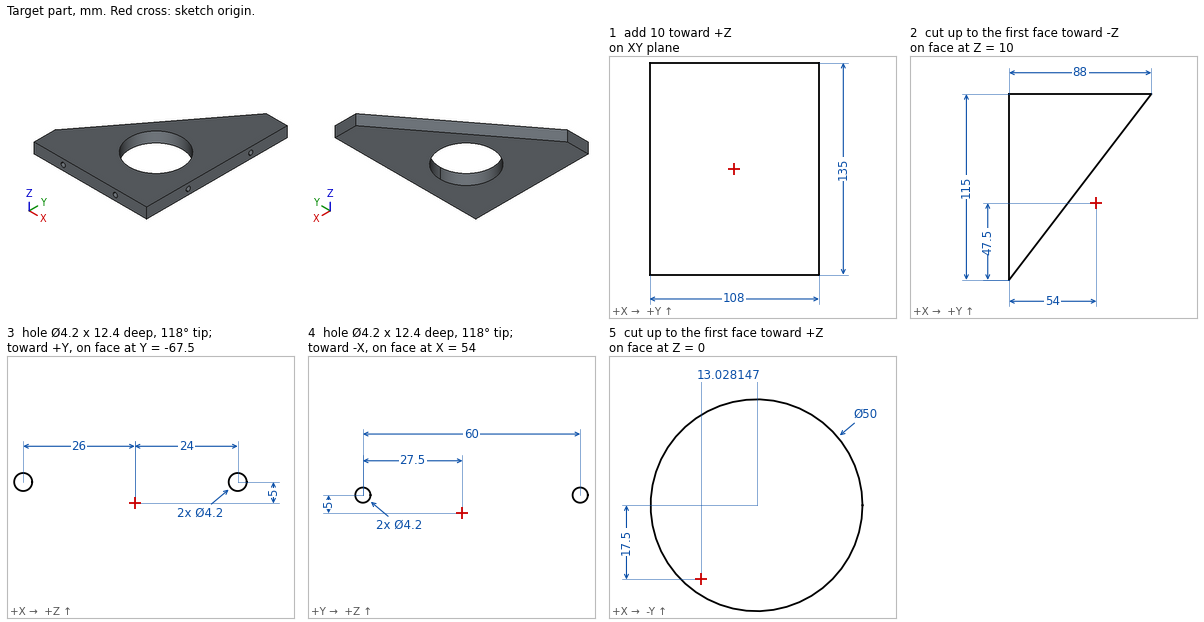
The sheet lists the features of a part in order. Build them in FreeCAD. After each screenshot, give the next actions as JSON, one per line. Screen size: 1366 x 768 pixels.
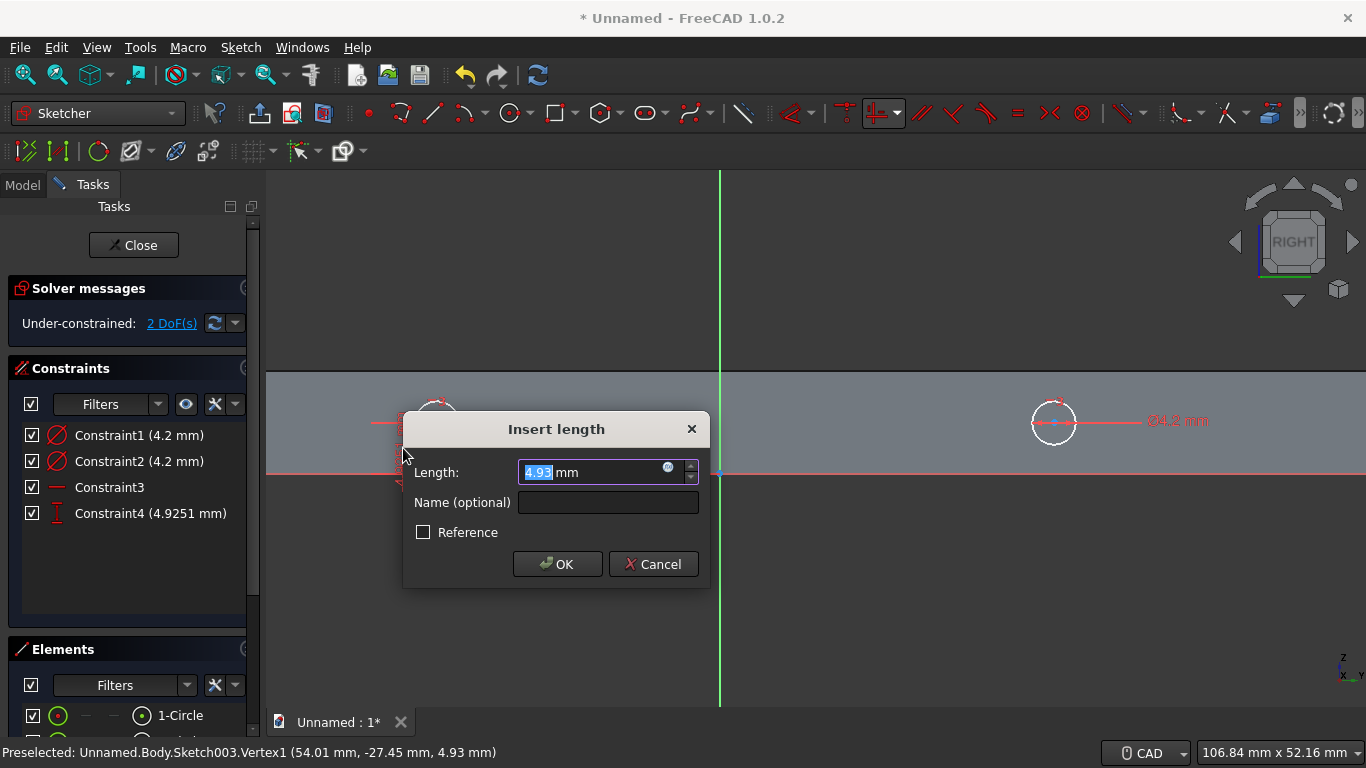
{"action": "type", "text": "5"}
{"action": "key", "text": "Return"}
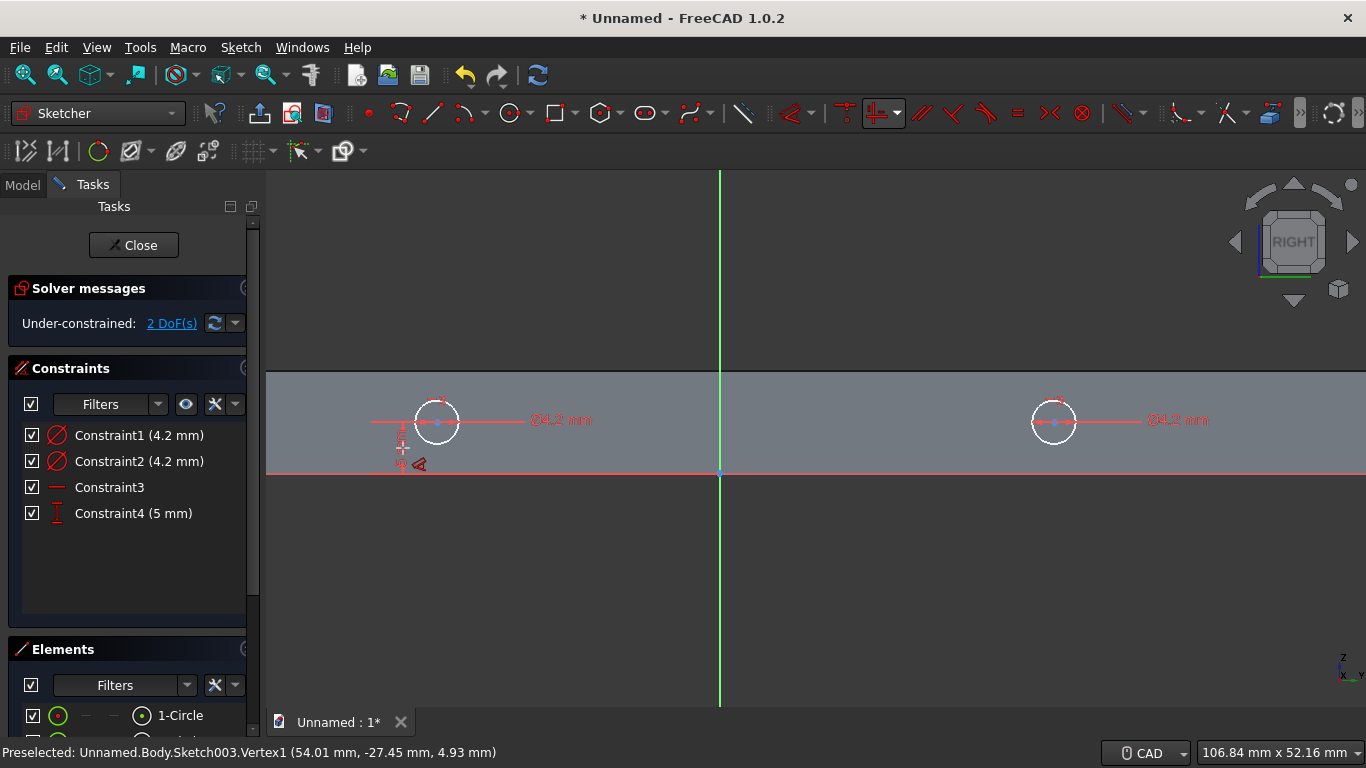
{"action": "left_click", "coordinate": [437, 422]}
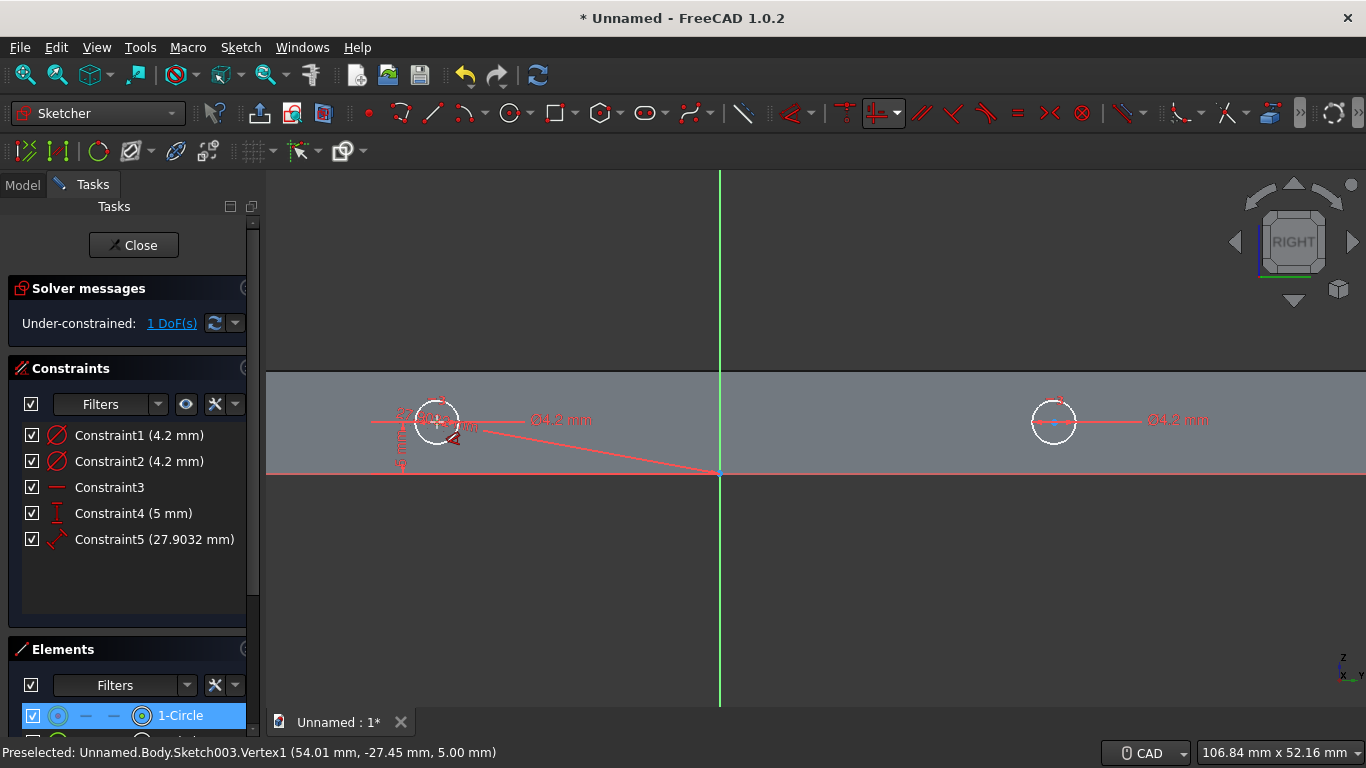
{"action": "left_click", "coordinate": [1054, 422]}
{"action": "left_click", "coordinate": [745, 388]}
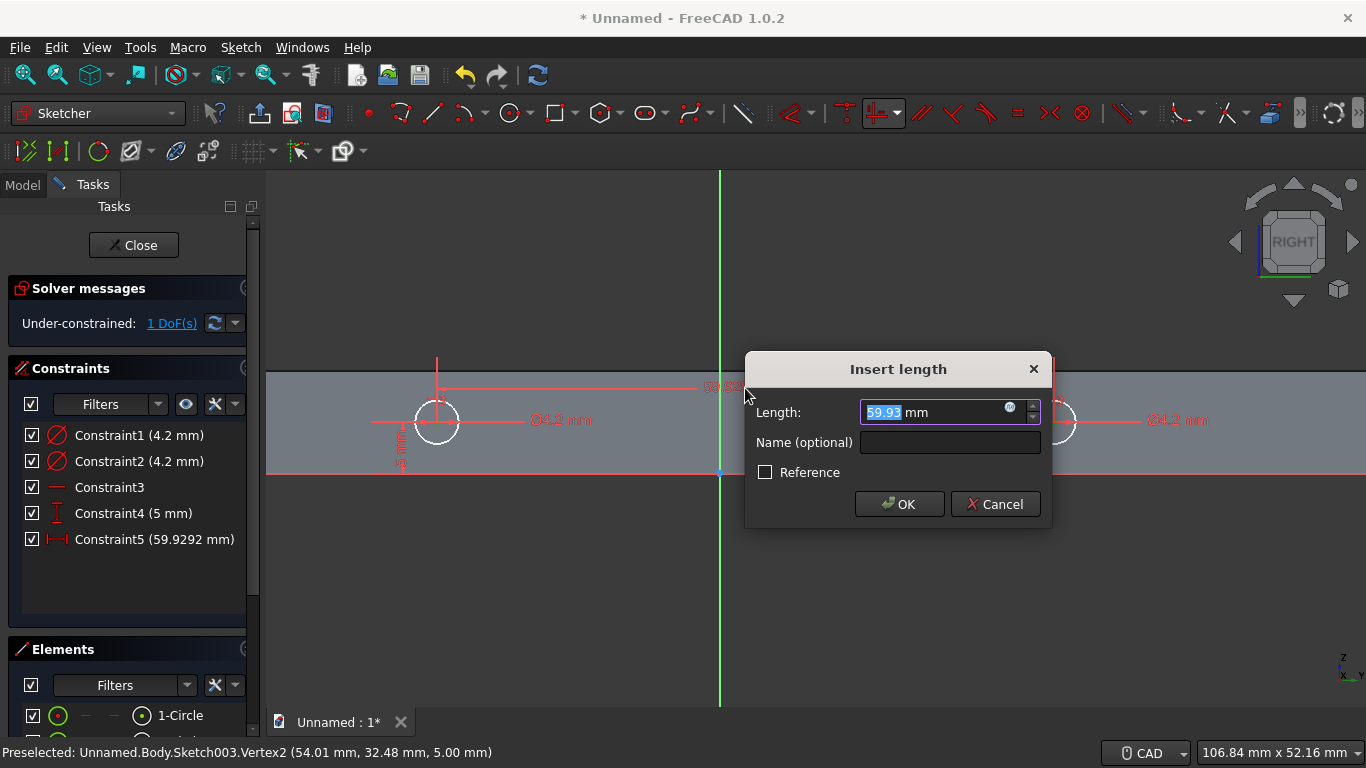
{"action": "type", "text": "60"}
{"action": "key", "text": "Return"}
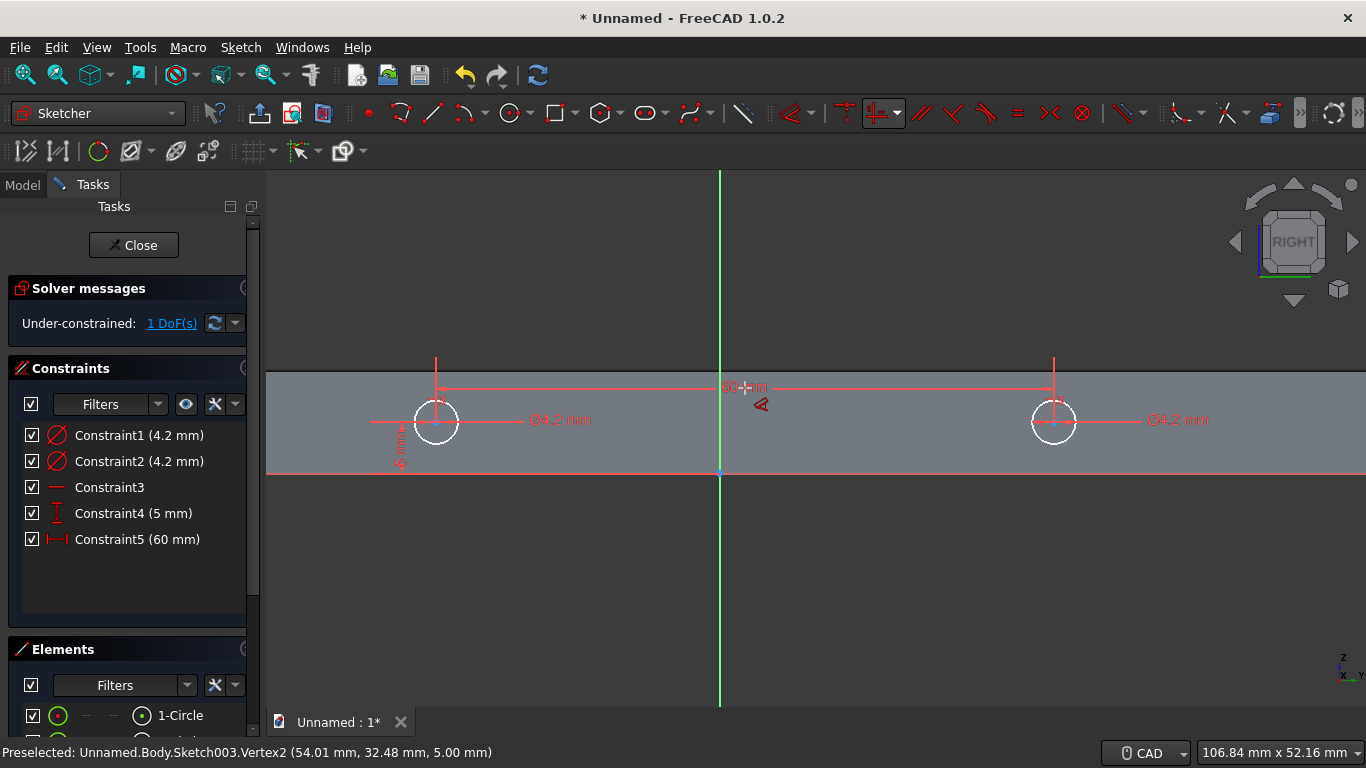
{"action": "left_click", "coordinate": [436, 422]}
{"action": "left_click", "coordinate": [578, 508]}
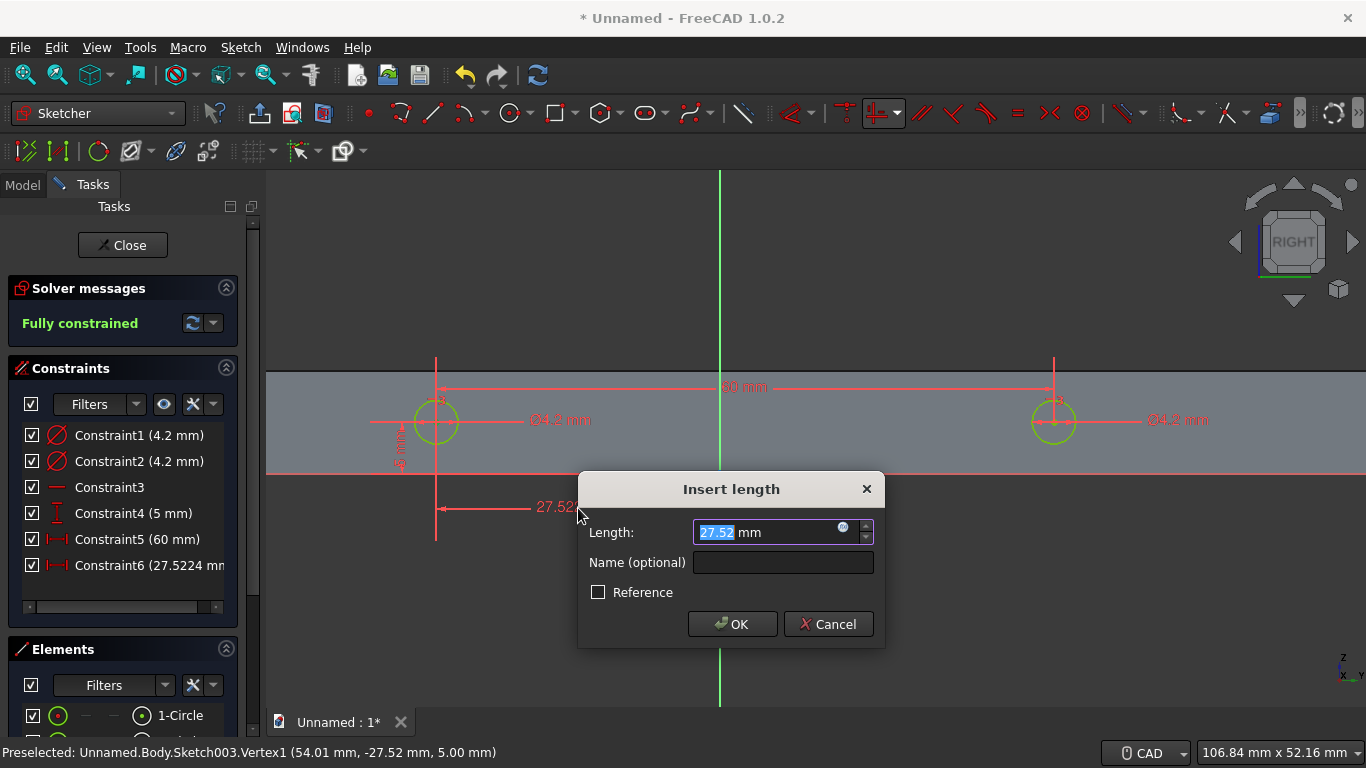
{"action": "type", "text": "27.5"}
{"action": "key", "text": "Return"}
{"action": "key", "text": "Escape"}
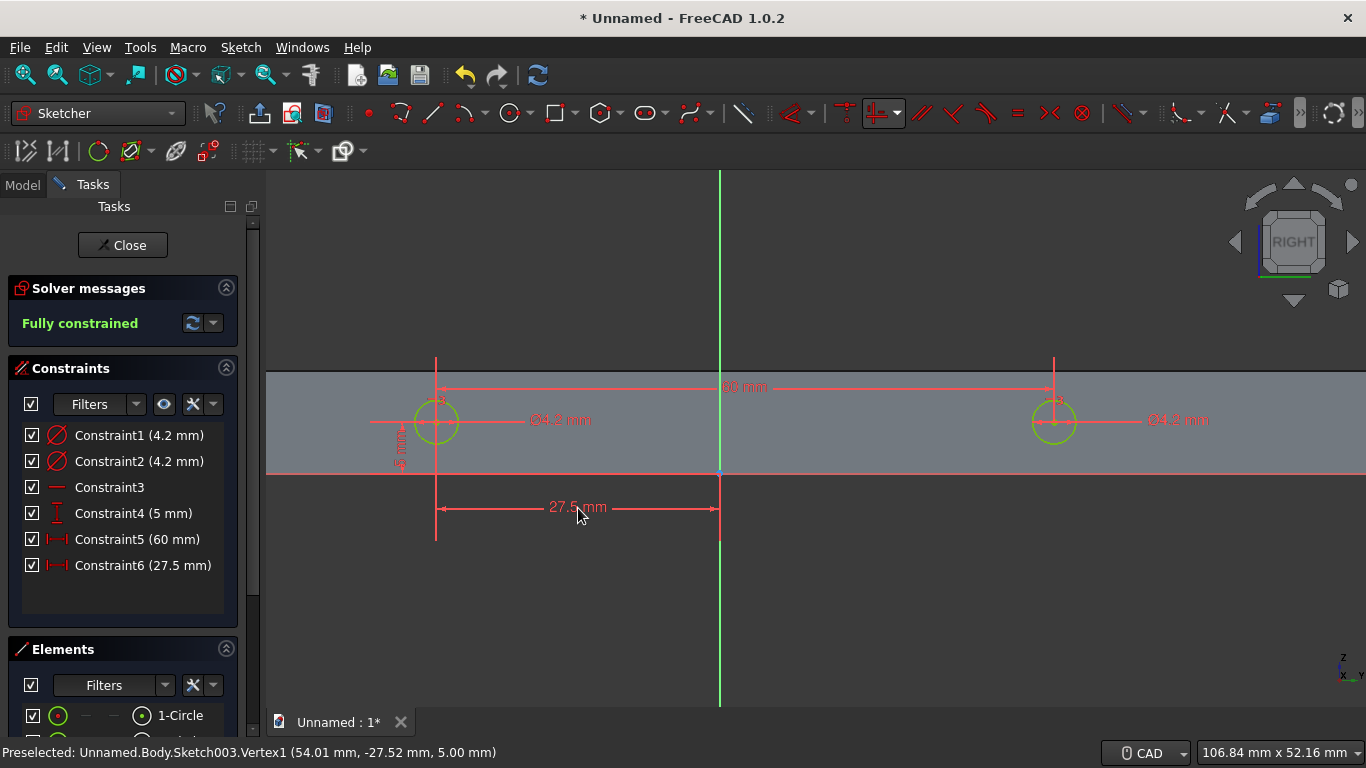
{"action": "left_click", "coordinate": [123, 245]}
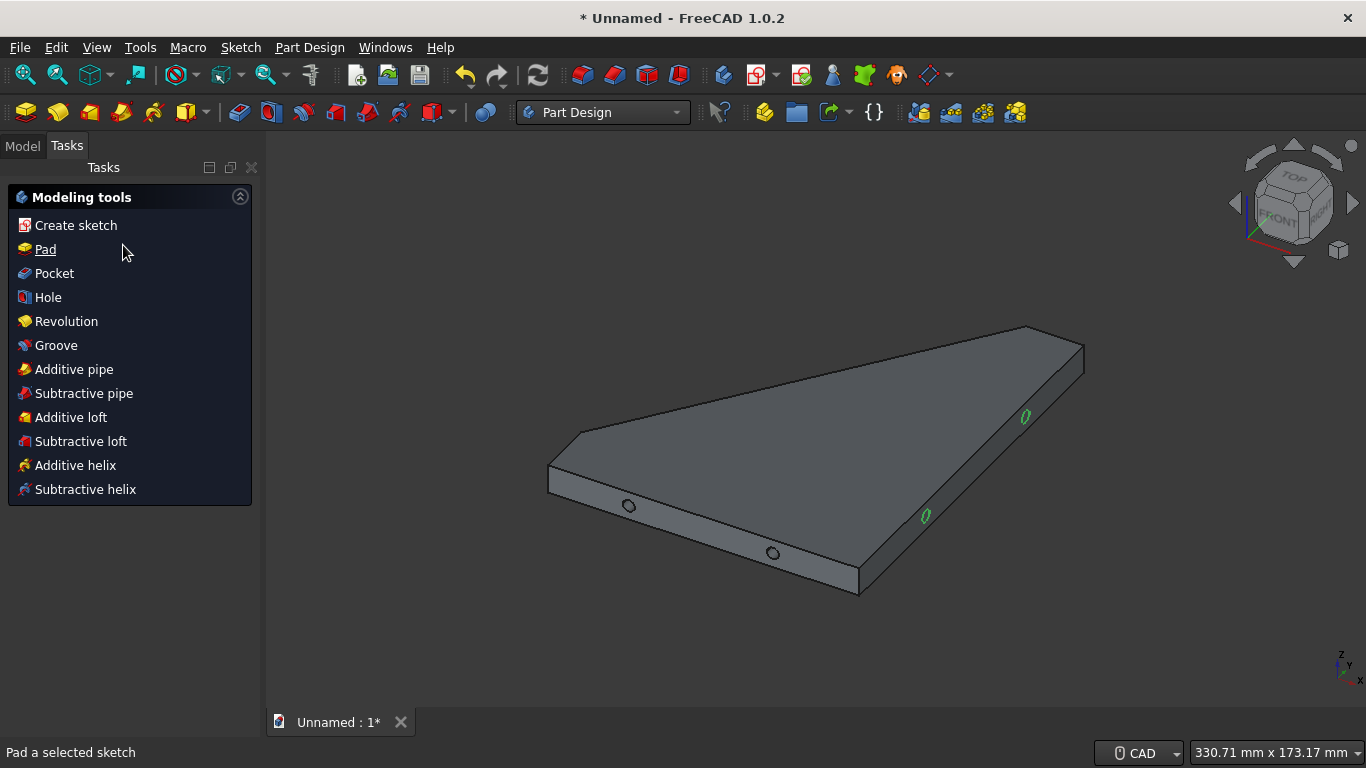
{"action": "left_click", "coordinate": [272, 112]}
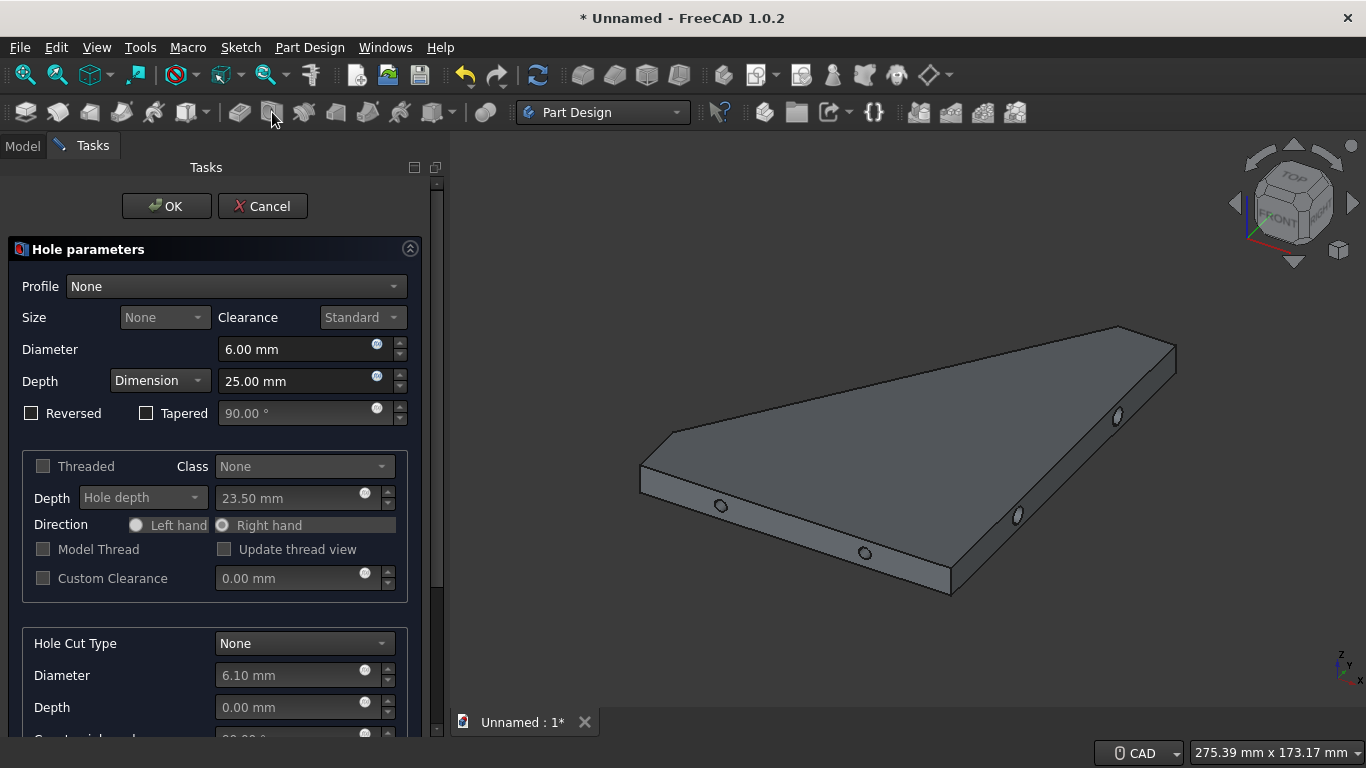
{"action": "triple_click", "coordinate": [305, 349]}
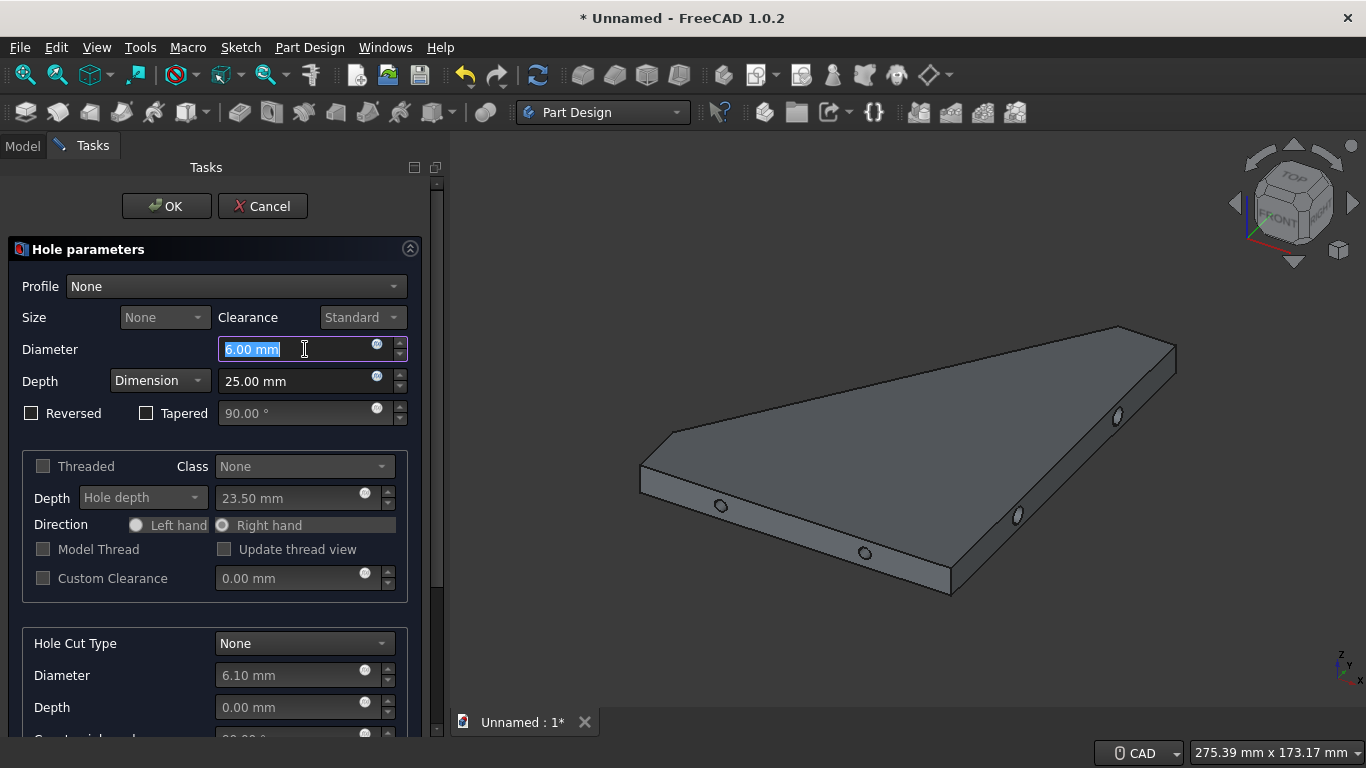
{"action": "type", "text": "4.2"}
{"action": "key", "text": "Tab"}